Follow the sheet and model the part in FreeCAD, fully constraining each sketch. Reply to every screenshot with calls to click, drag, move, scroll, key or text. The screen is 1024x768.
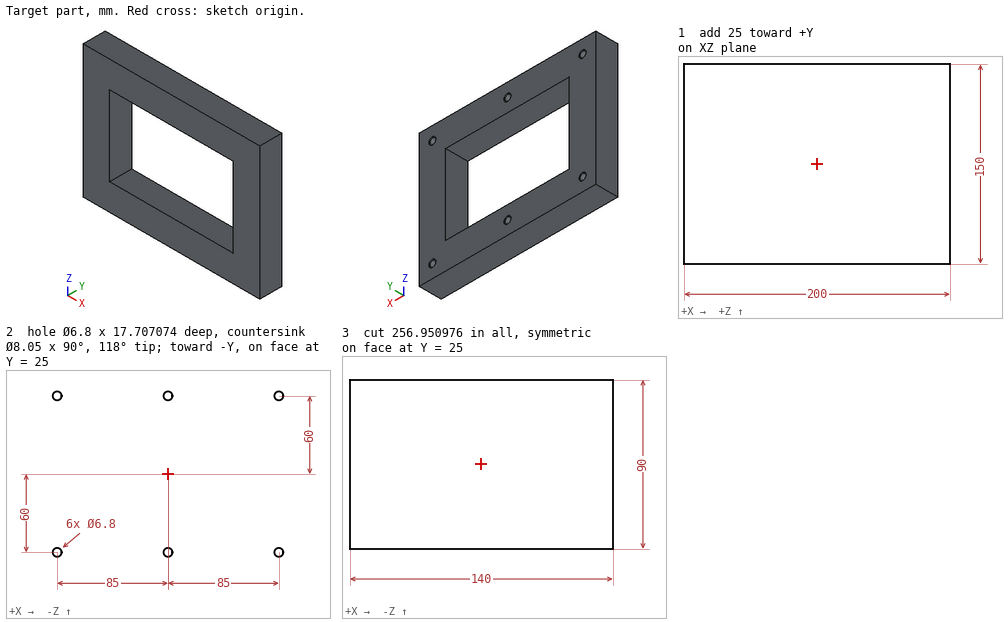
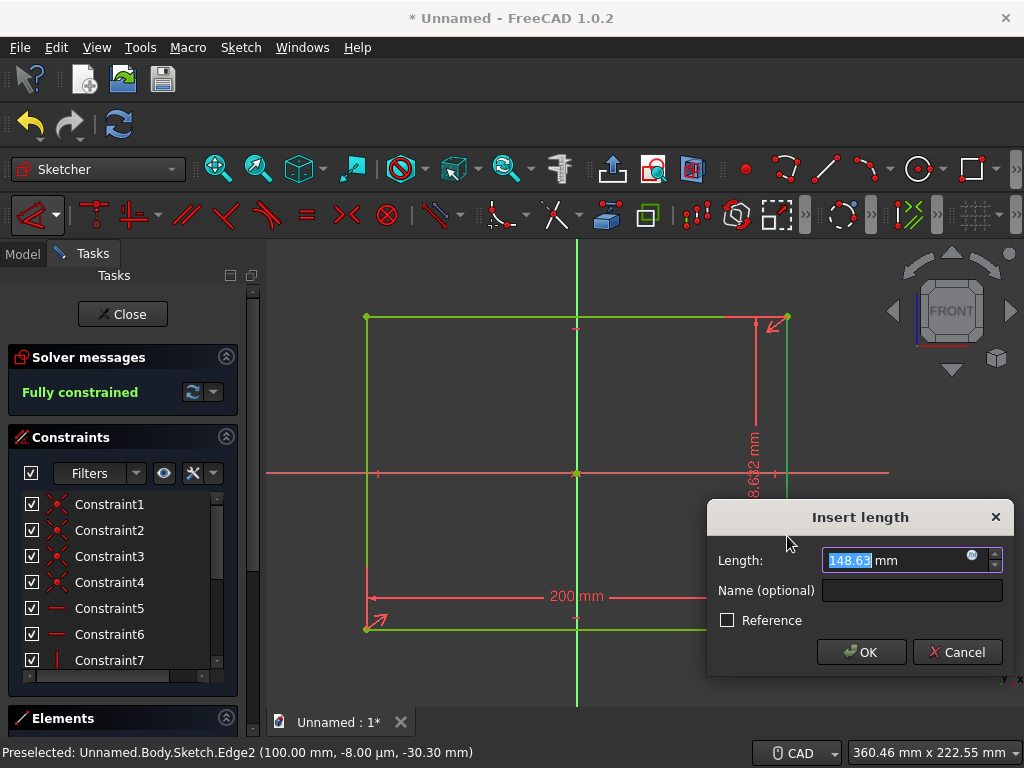
text(150)
key(Return)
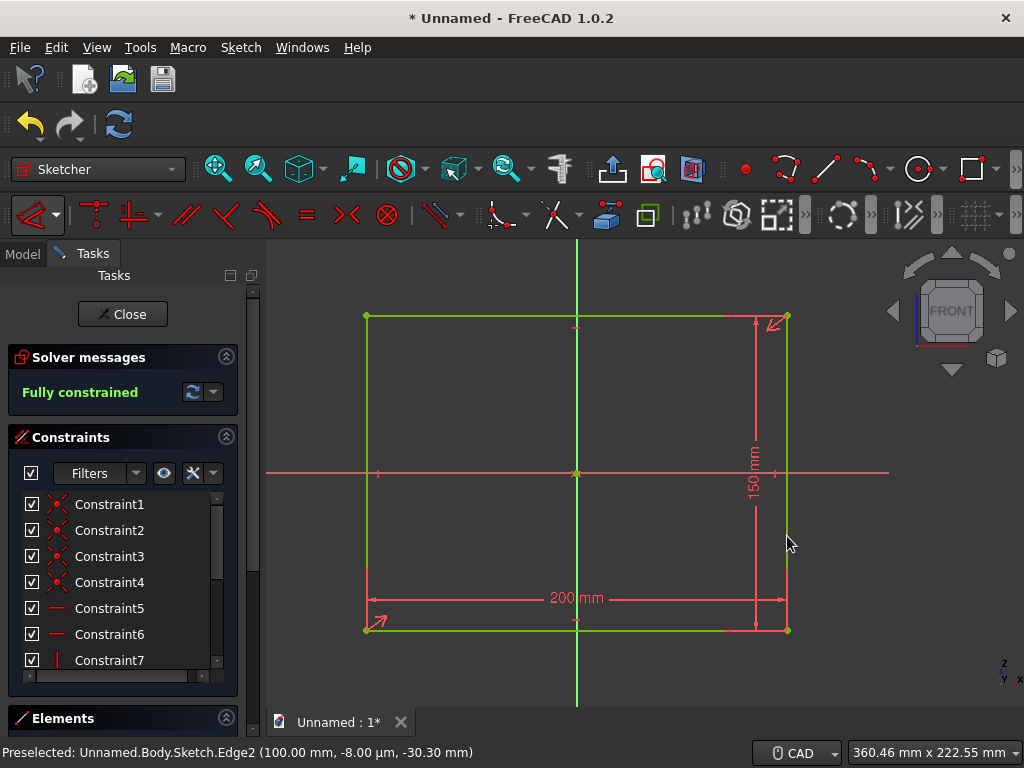
click(123, 314)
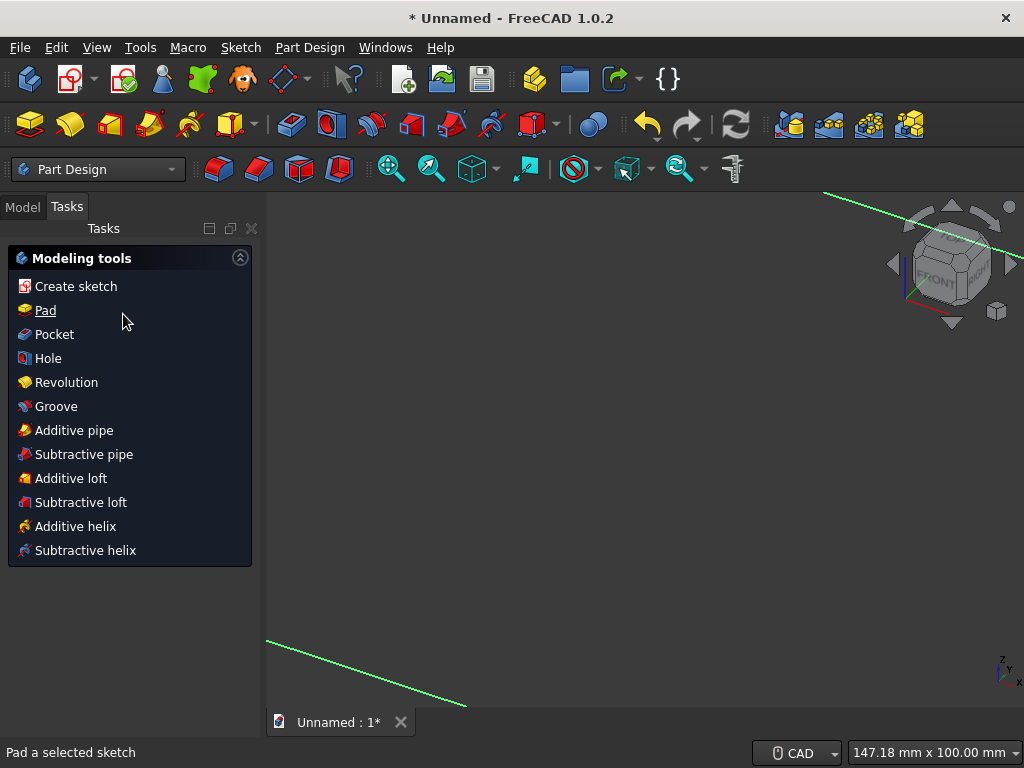
click(30, 124)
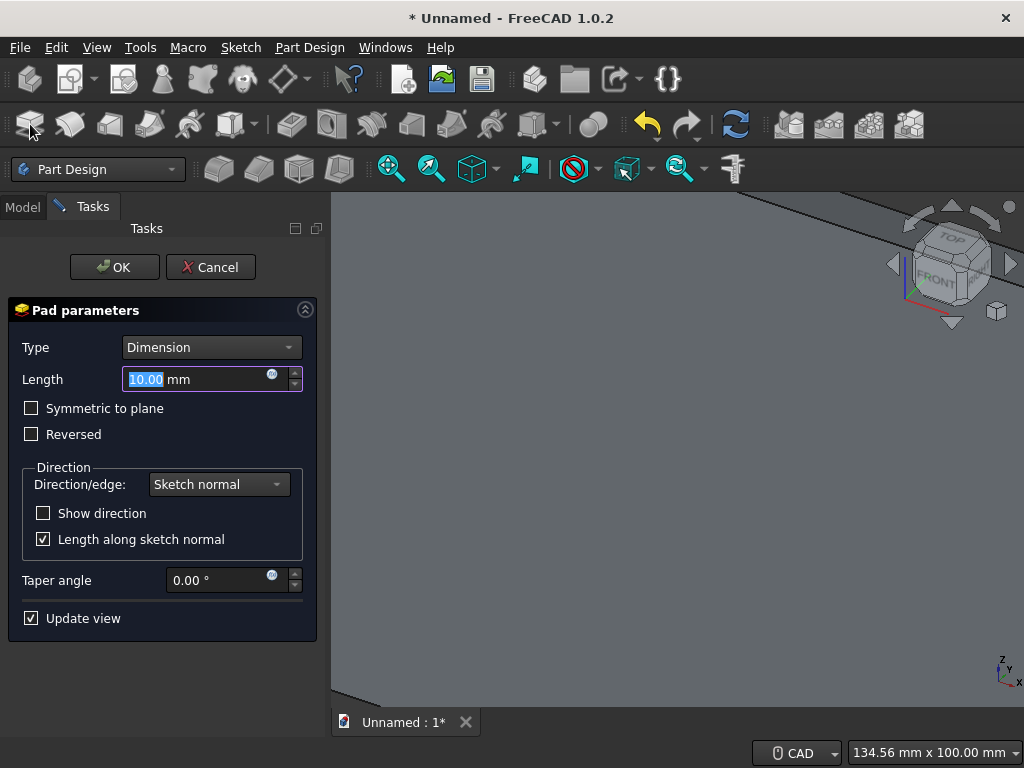
text(25)
key(Tab)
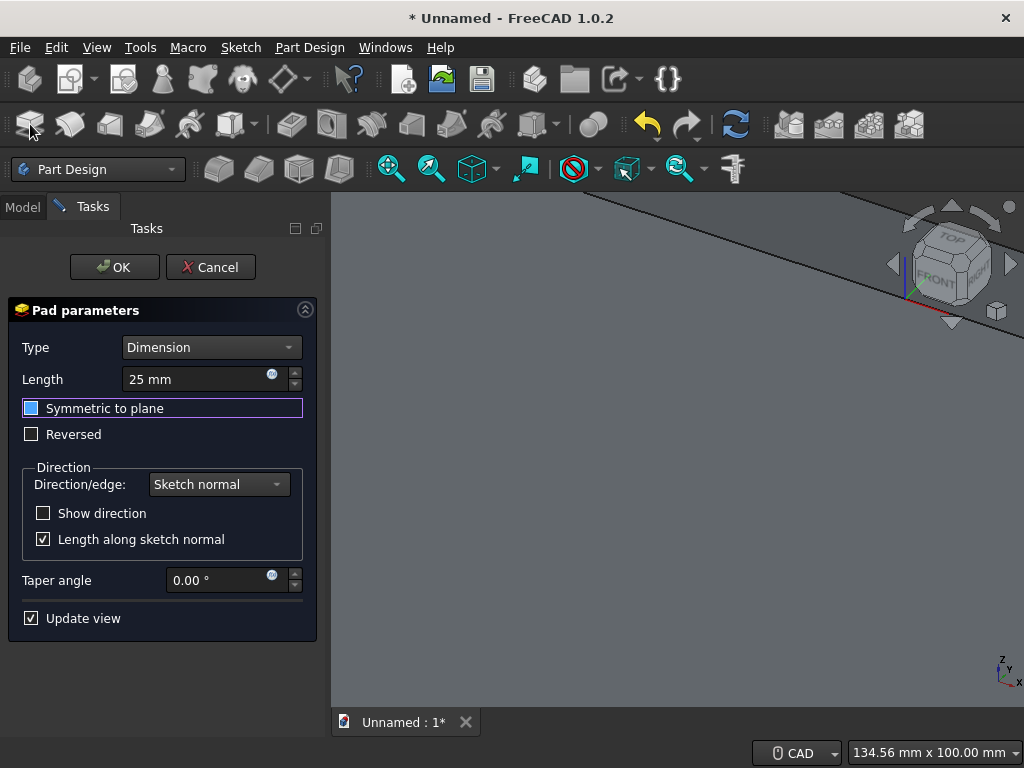
click(30, 434)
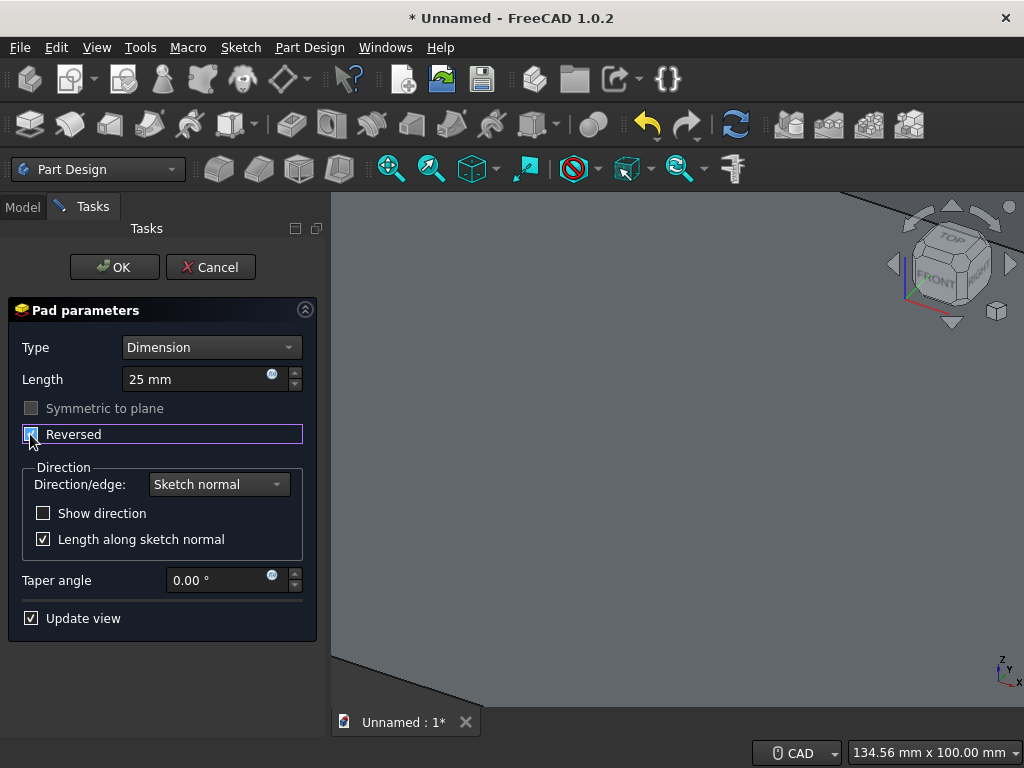
click(115, 267)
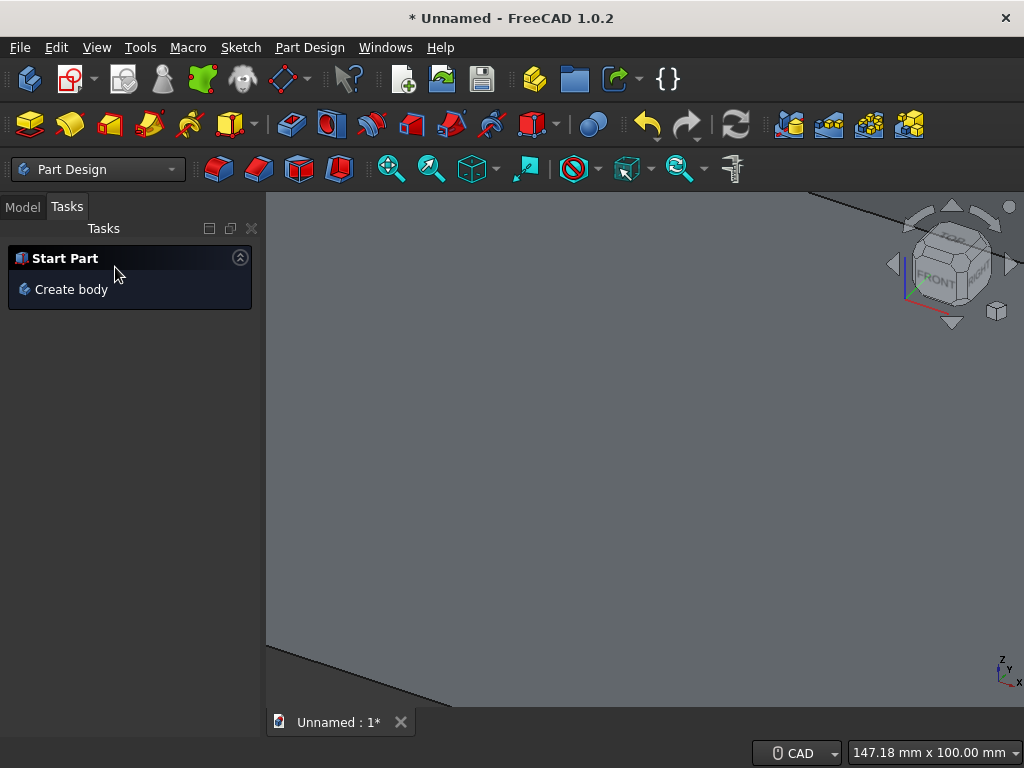
click(392, 170)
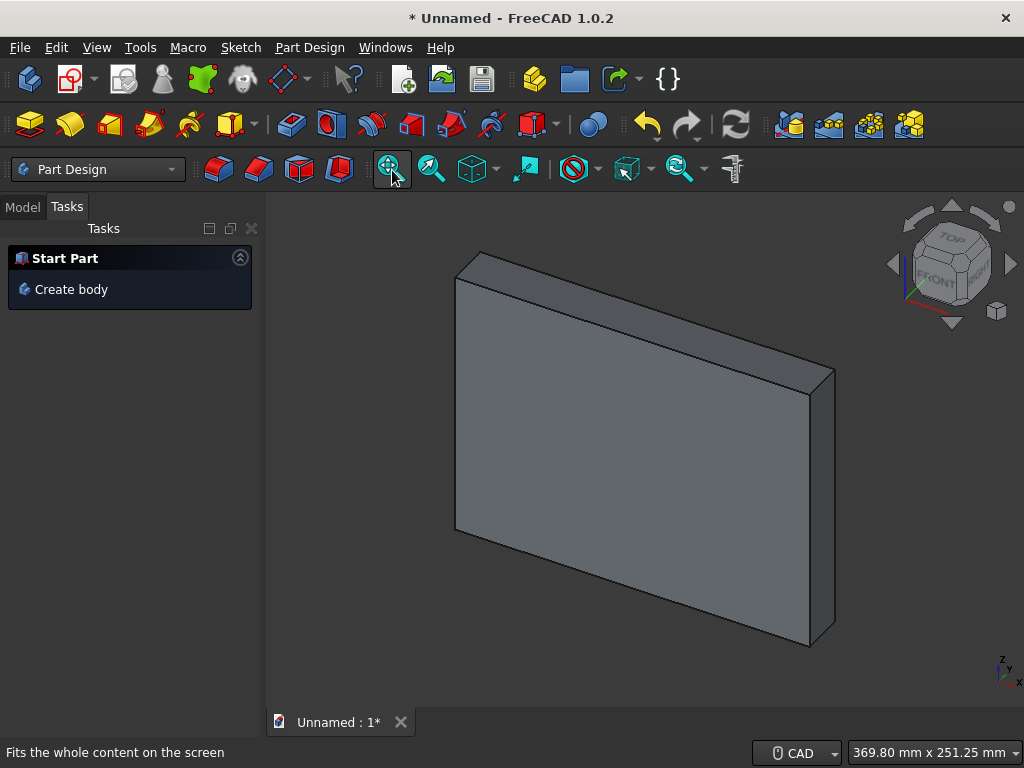
key(4)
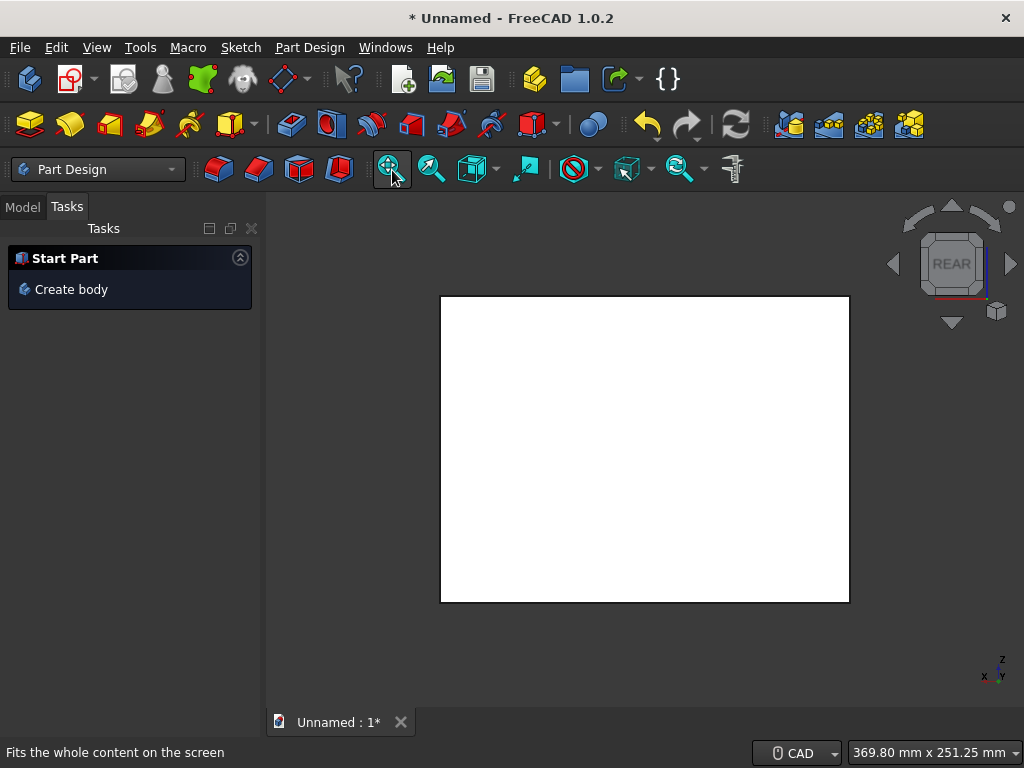
click(645, 448)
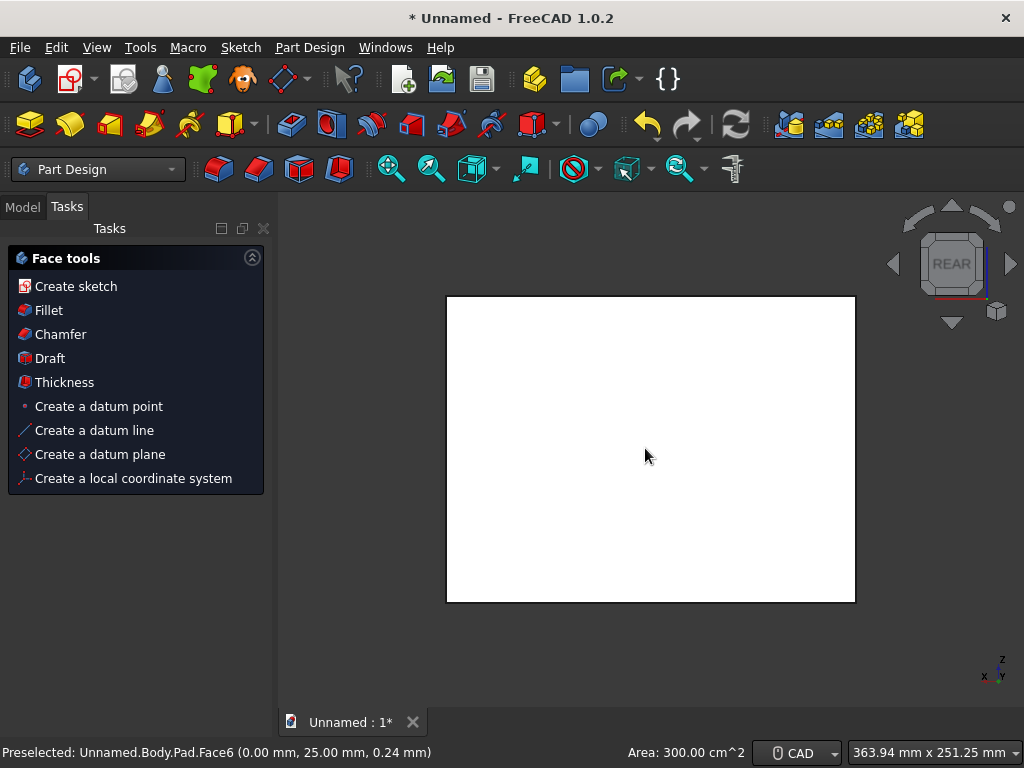
click(70, 80)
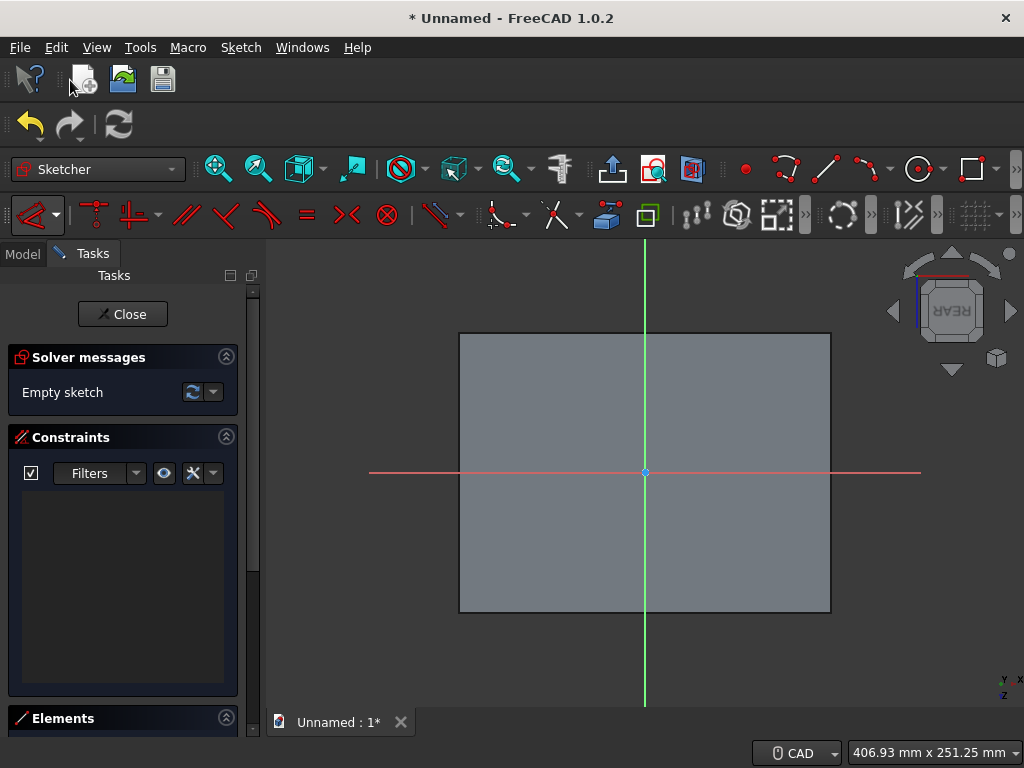
click(920, 170)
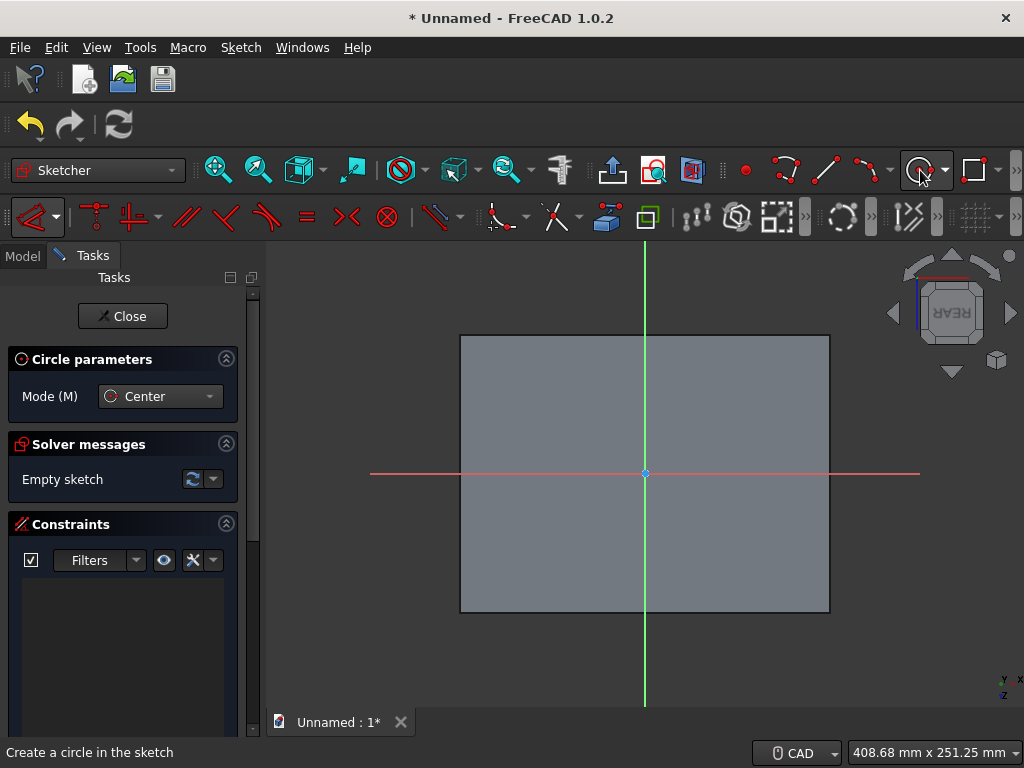
scroll(487, 585, up, 7)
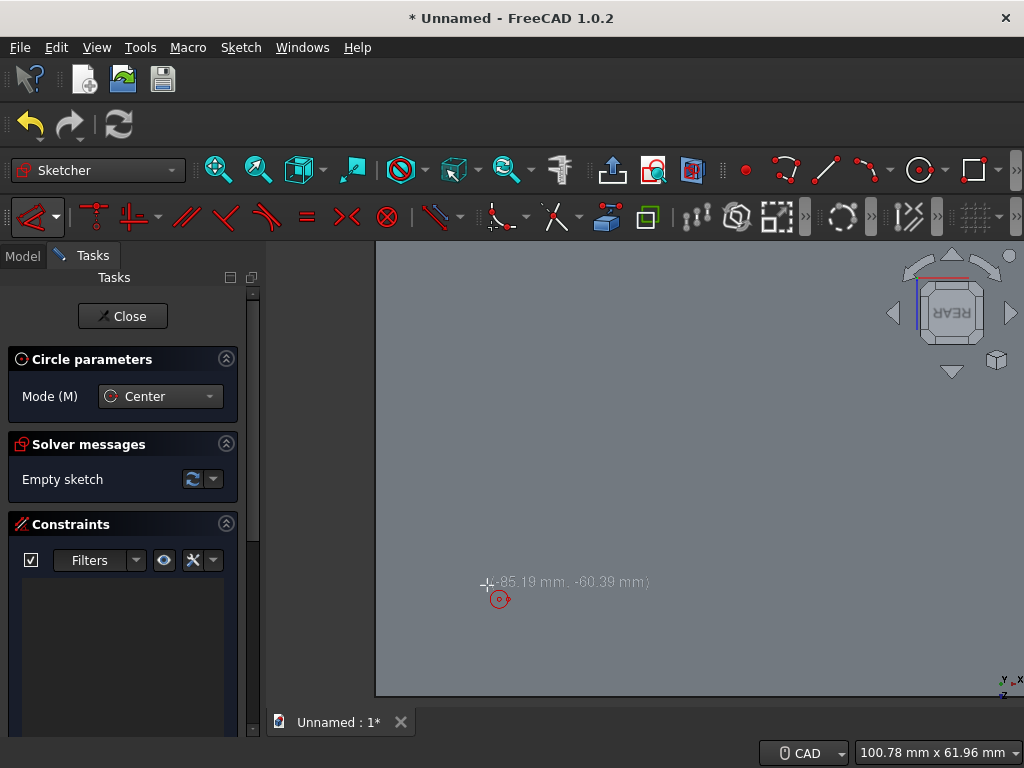
scroll(339, 621, down, 6)